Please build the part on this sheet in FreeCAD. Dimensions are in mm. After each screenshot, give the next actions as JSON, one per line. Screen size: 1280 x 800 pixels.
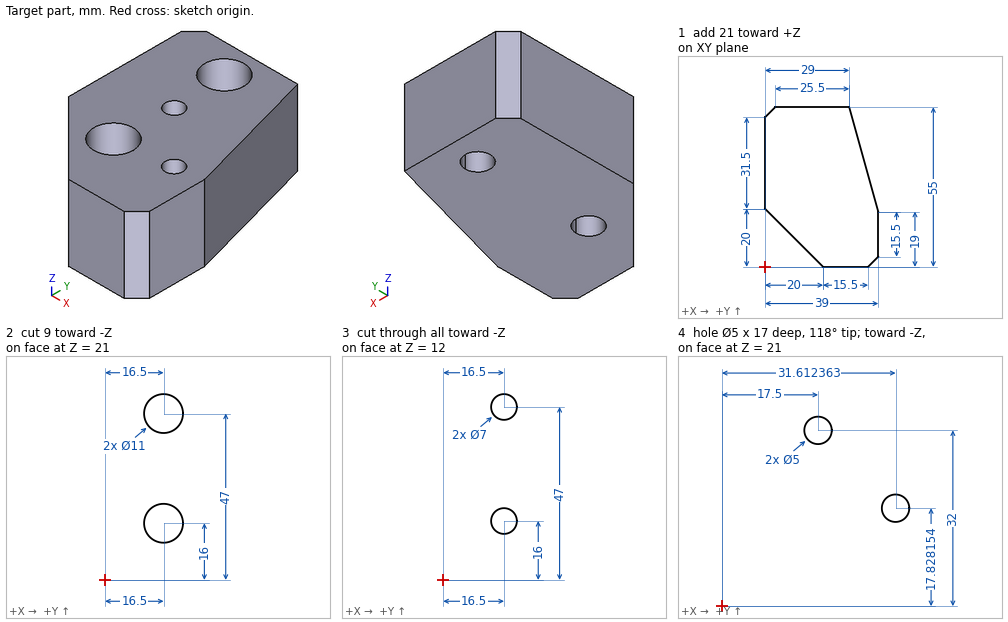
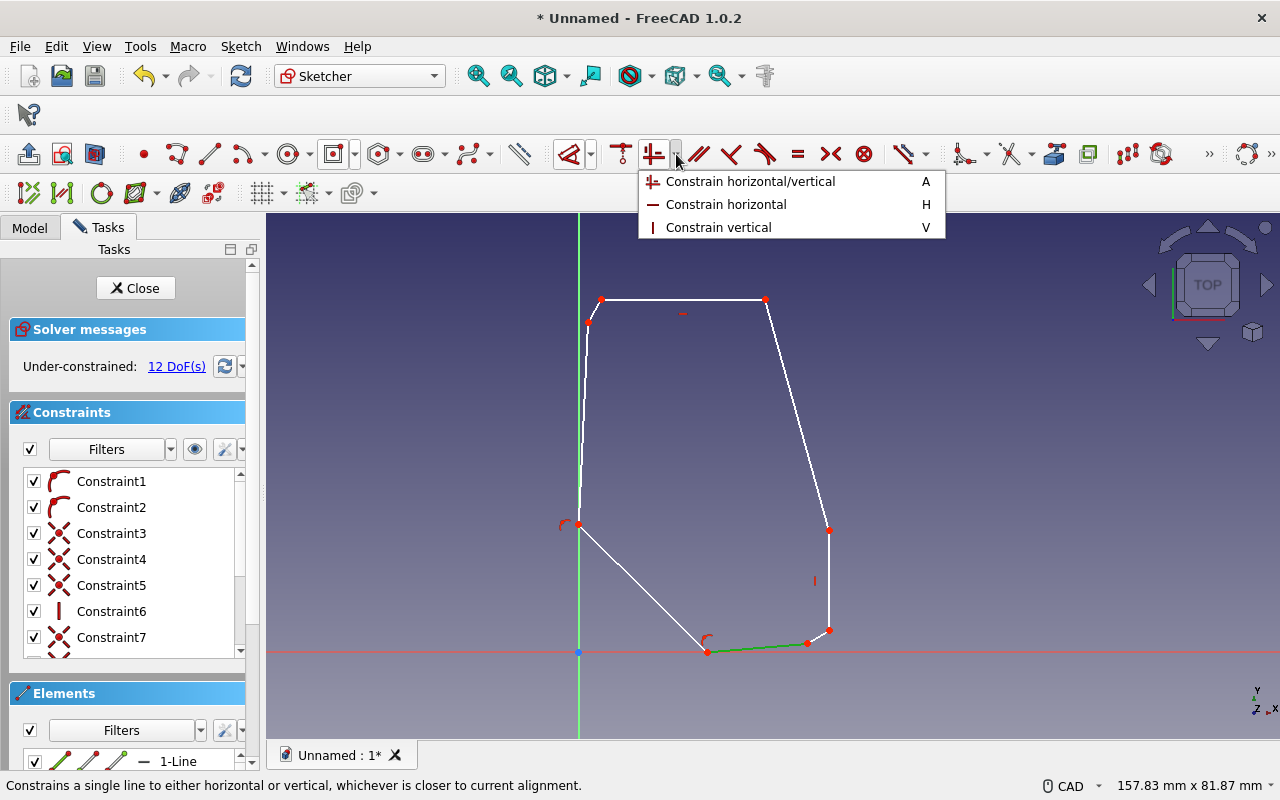
{"action": "left_click", "coordinate": [792, 204]}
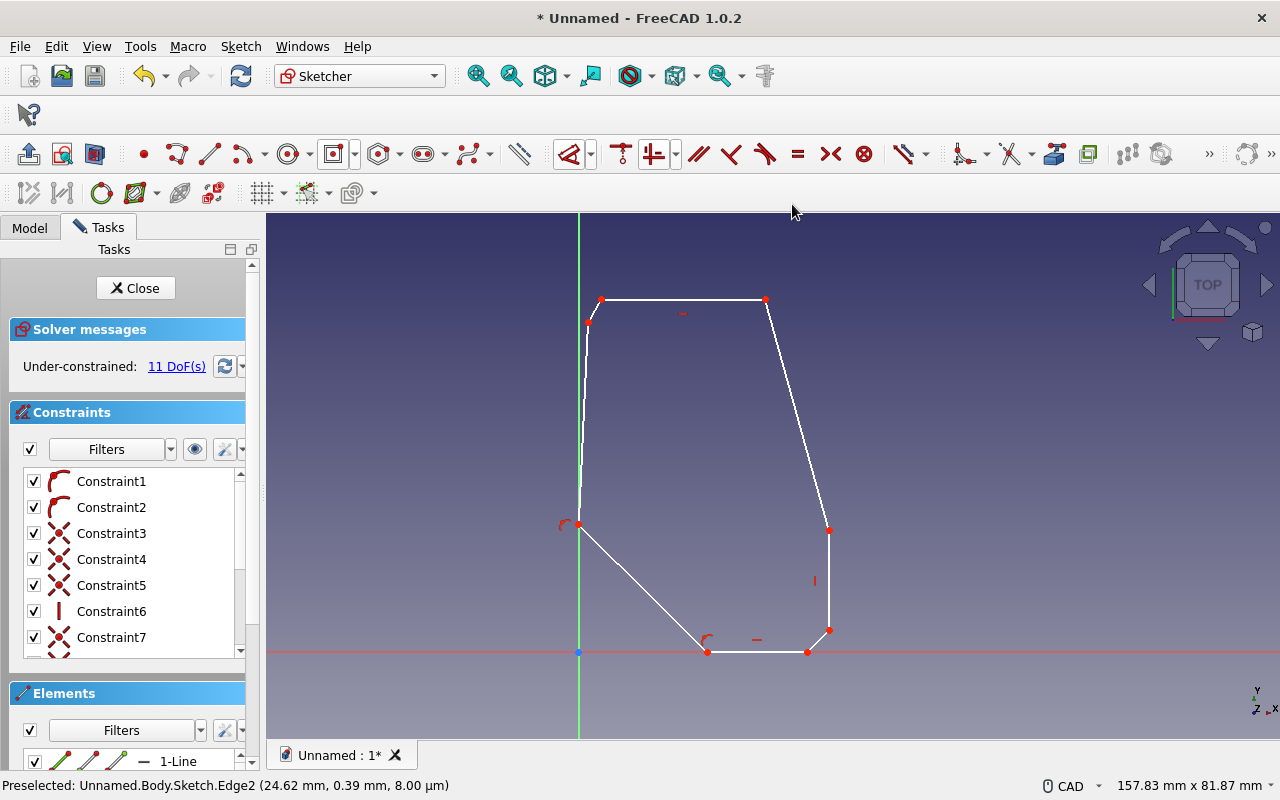
{"action": "left_click", "coordinate": [582, 464]}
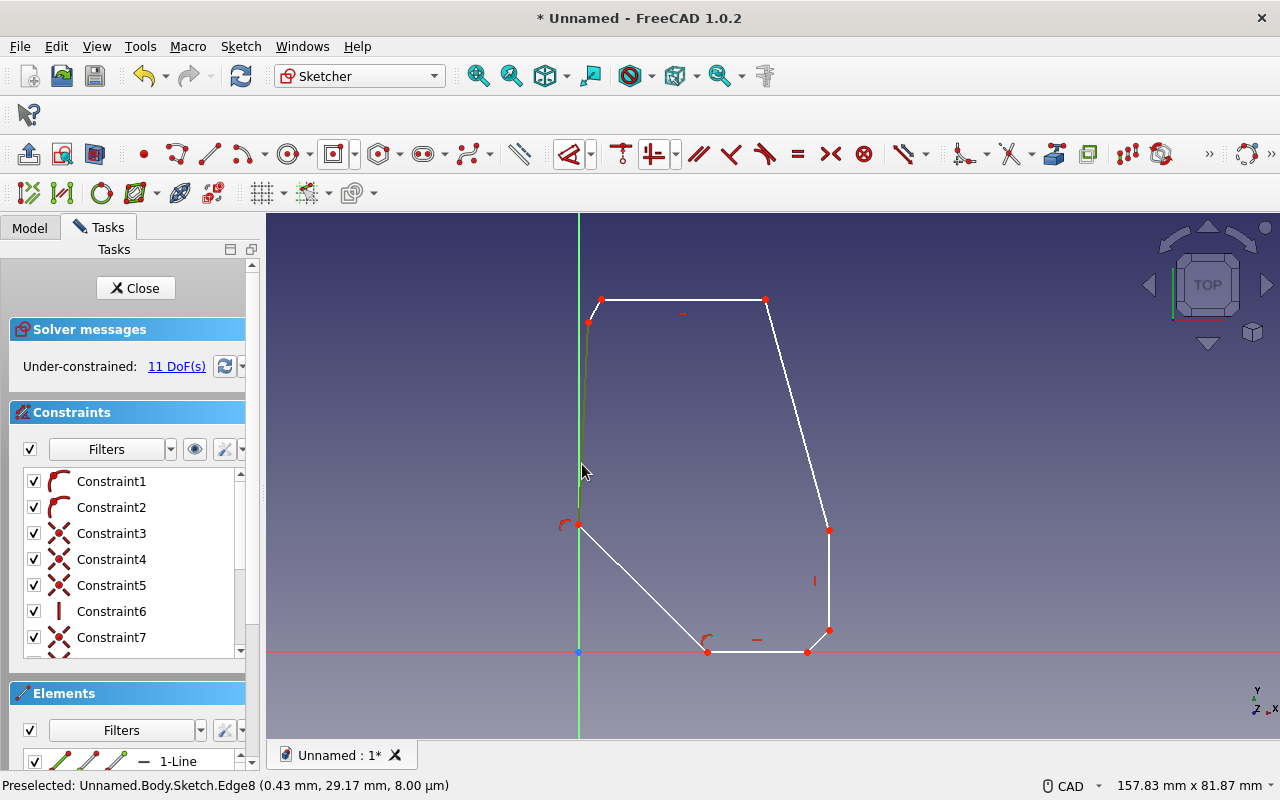
{"action": "left_click", "coordinate": [676, 154]}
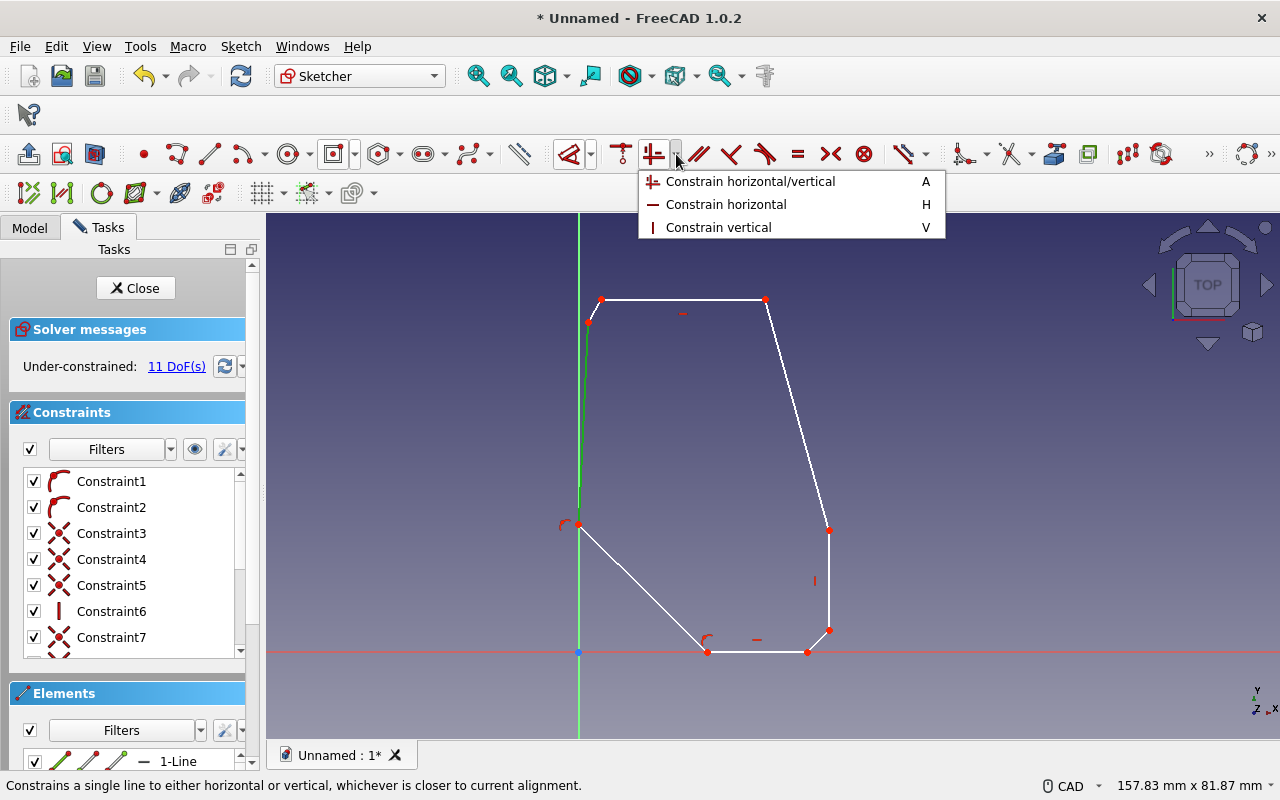
{"action": "left_click", "coordinate": [792, 228]}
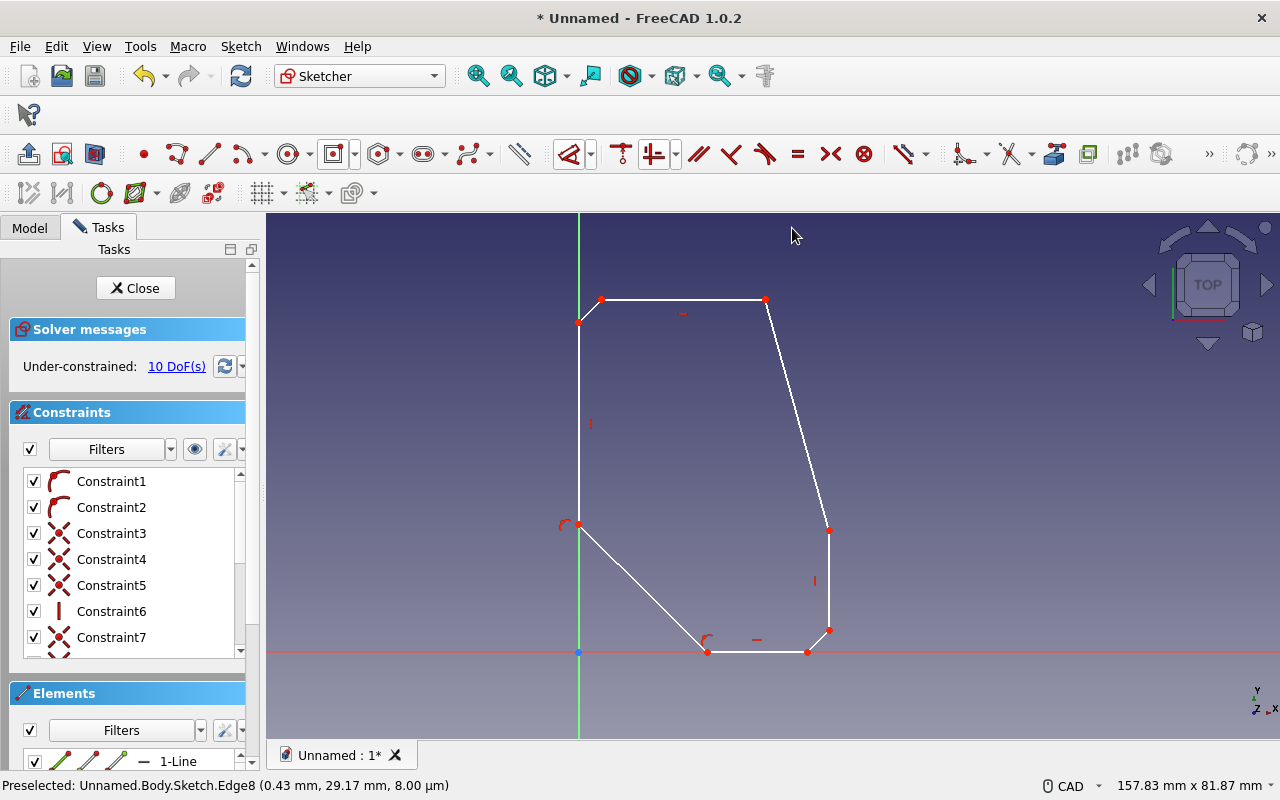
{"action": "left_click", "coordinate": [579, 525]}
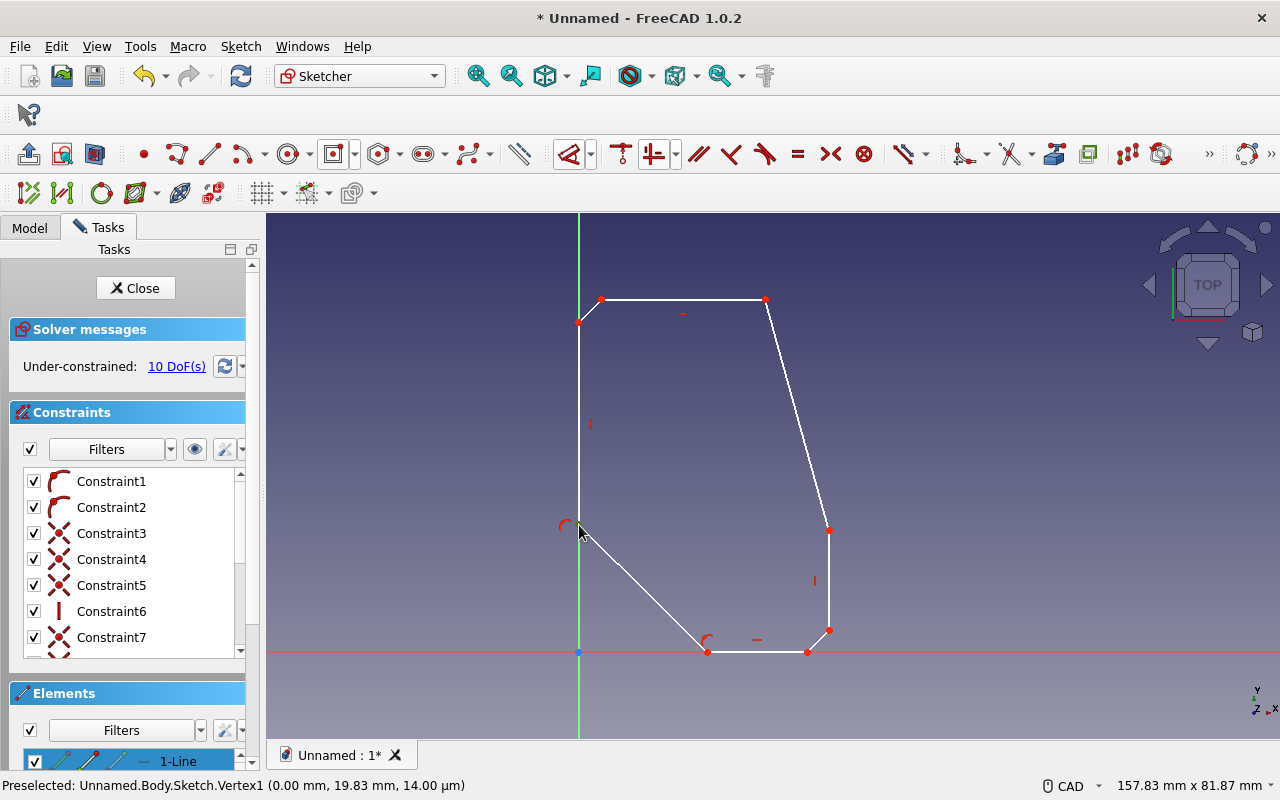
{"action": "key", "text": "i"}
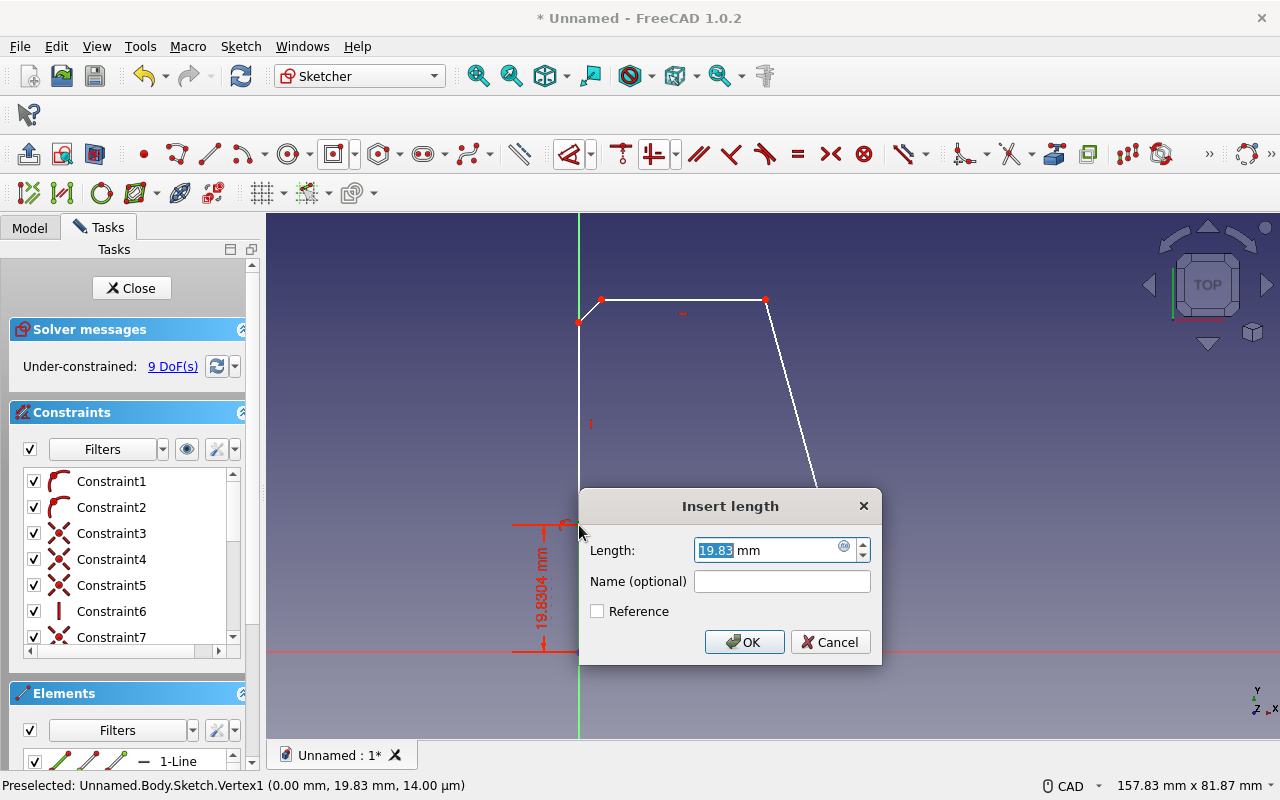
{"action": "type", "text": "20"}
{"action": "key", "text": "Return"}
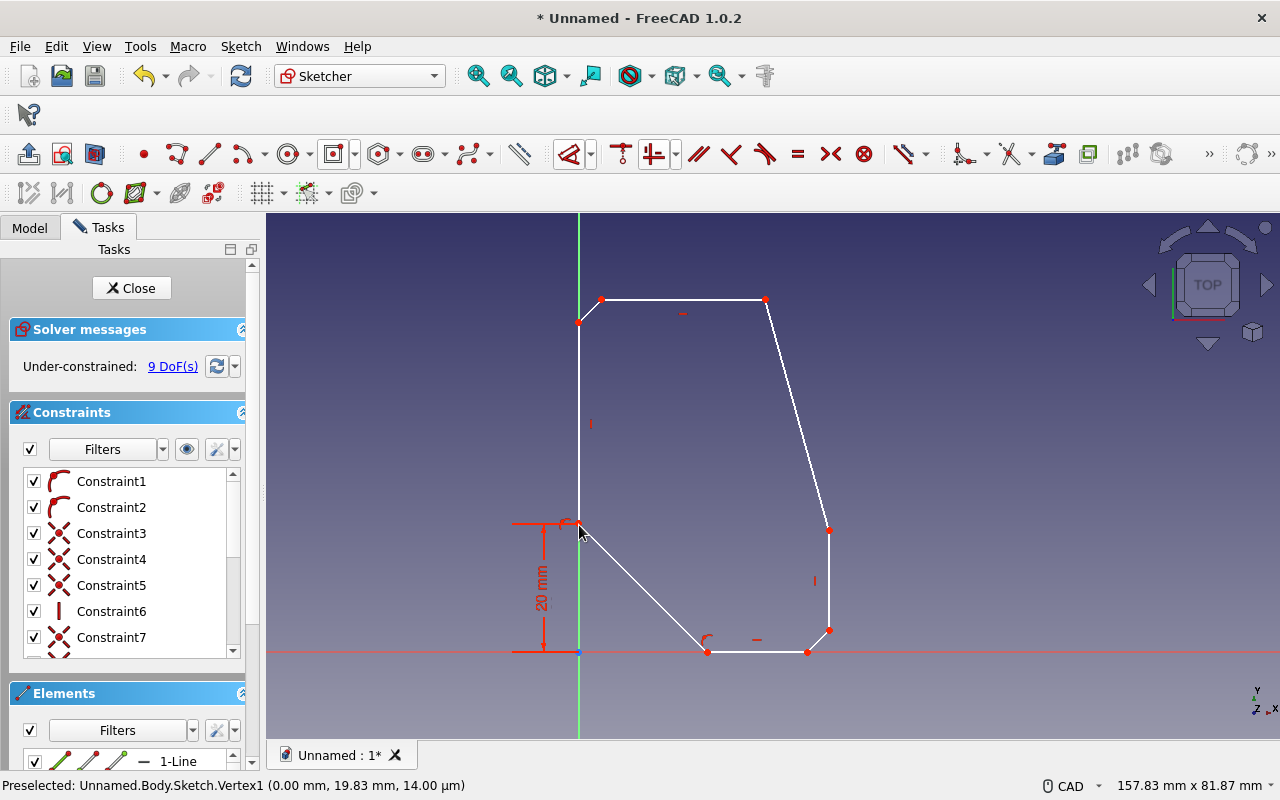
{"action": "left_click", "coordinate": [707, 652]}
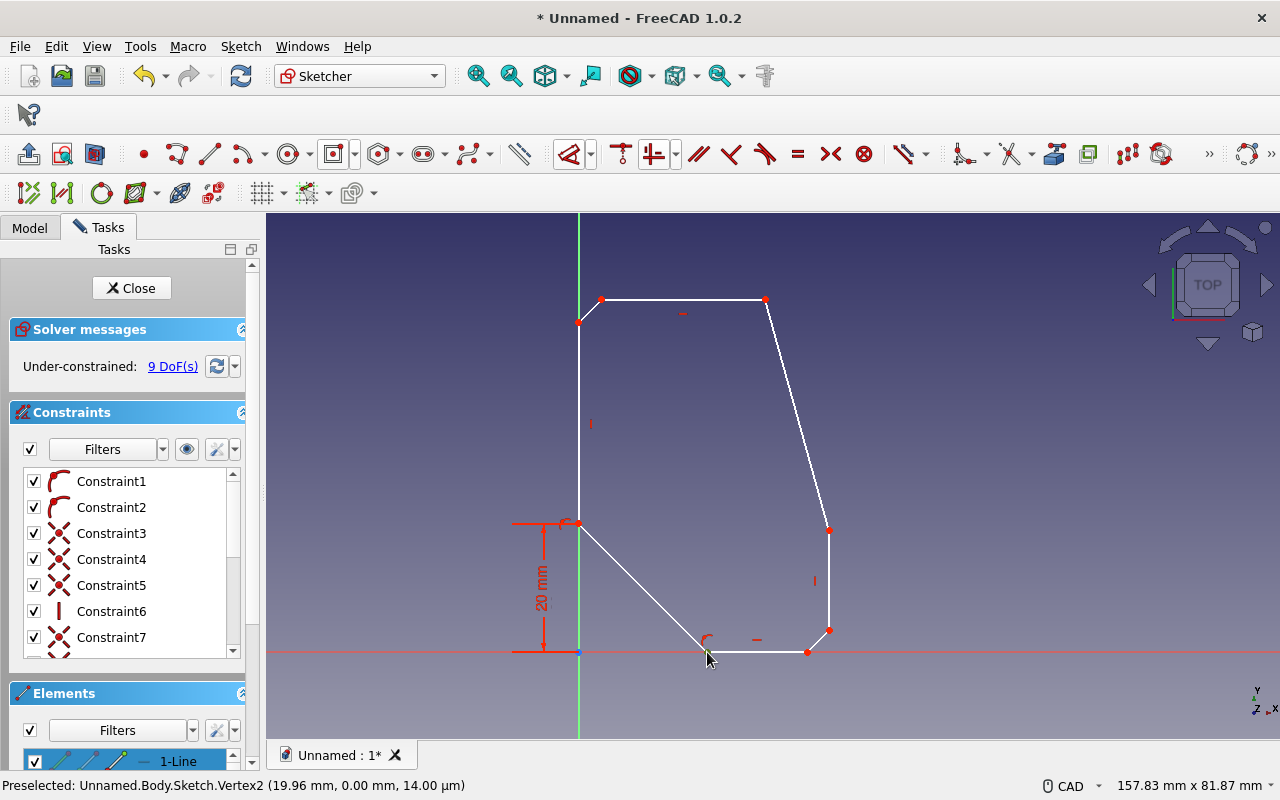
{"action": "key", "text": "l"}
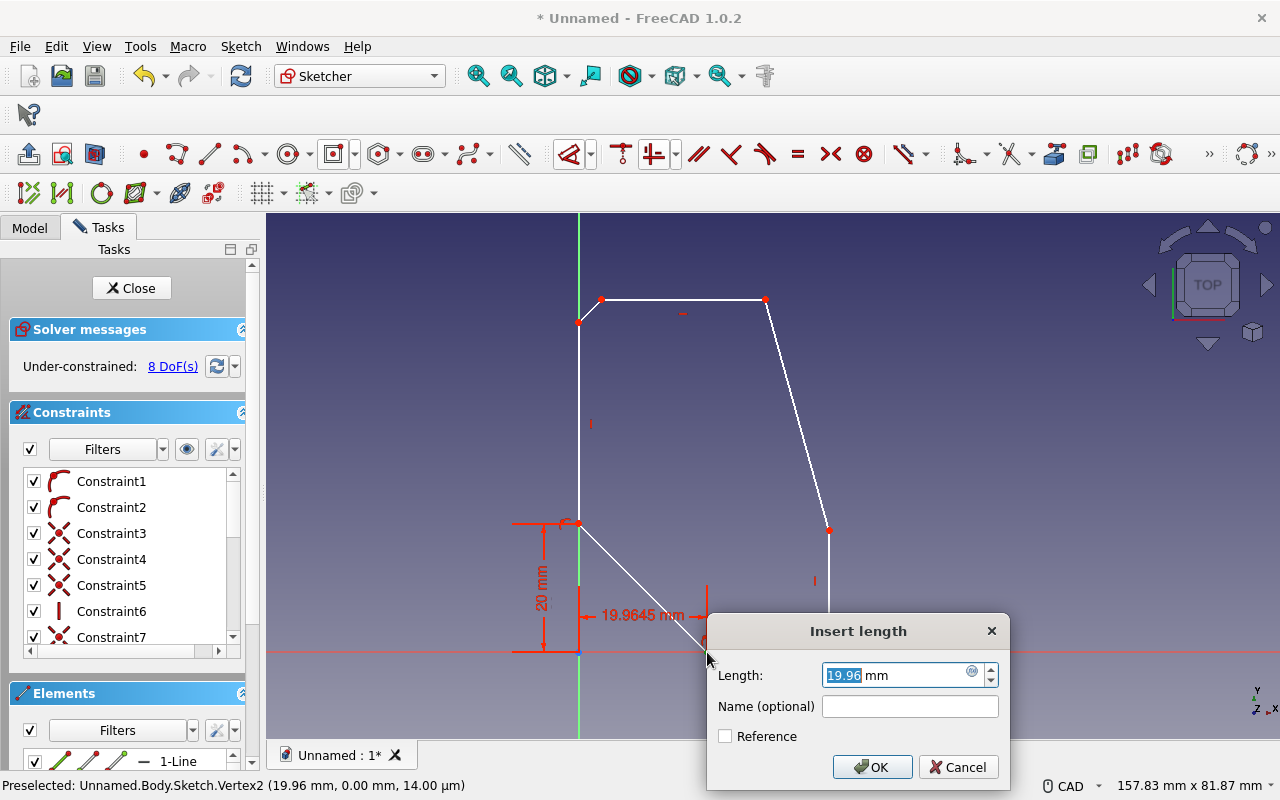
{"action": "type", "text": "20"}
{"action": "key", "text": "Return"}